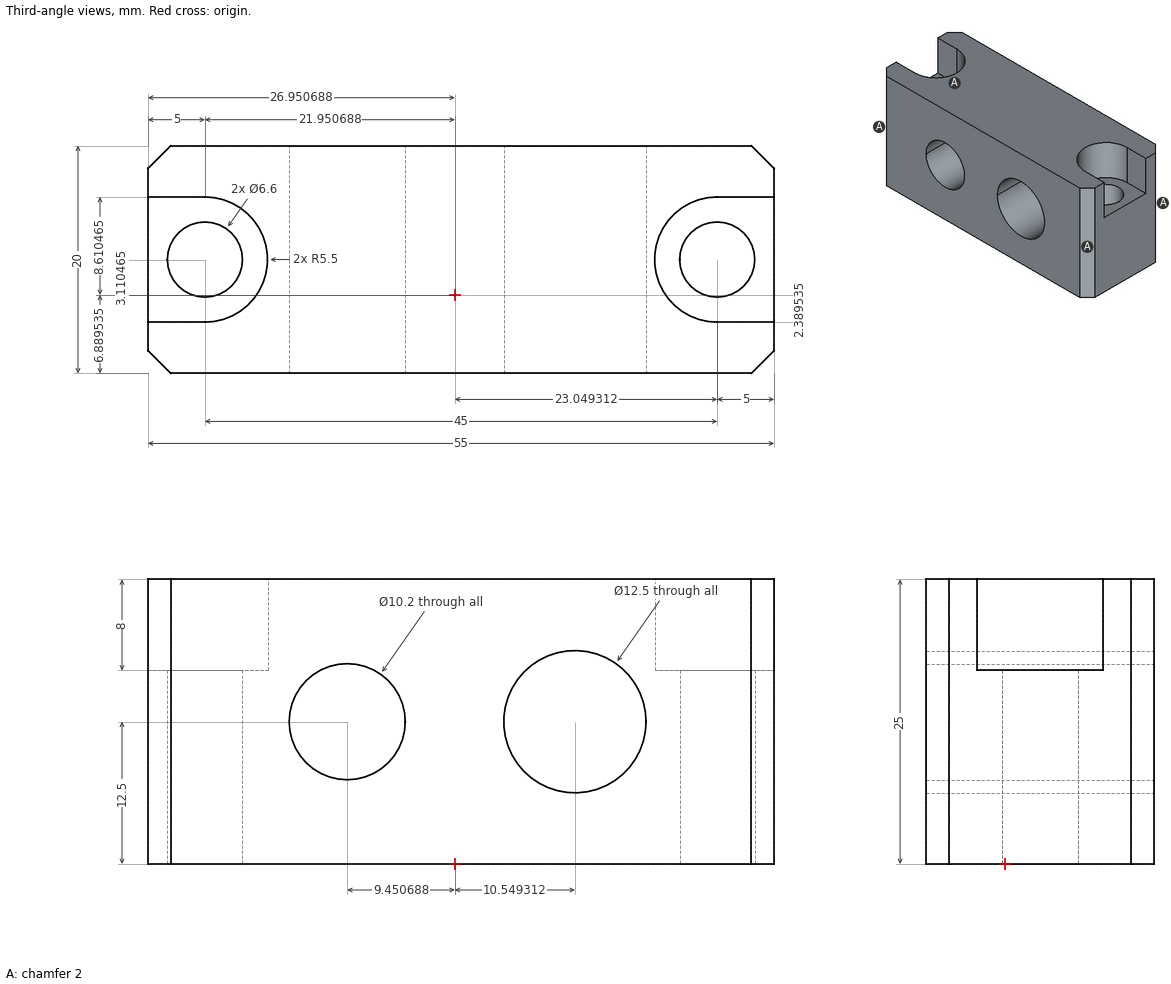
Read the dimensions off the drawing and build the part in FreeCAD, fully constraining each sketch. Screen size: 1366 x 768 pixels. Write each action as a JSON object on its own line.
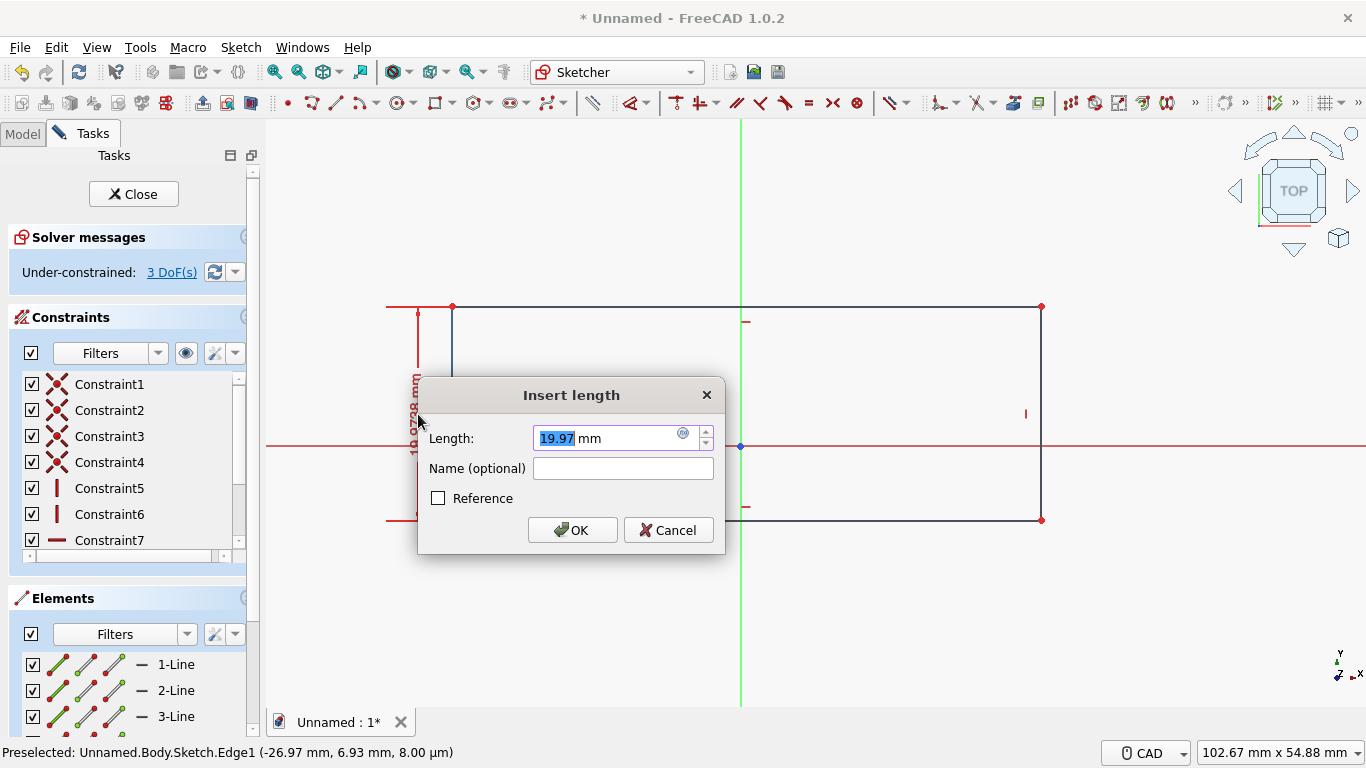
{"action": "type", "text": "20"}
{"action": "key", "text": "Return"}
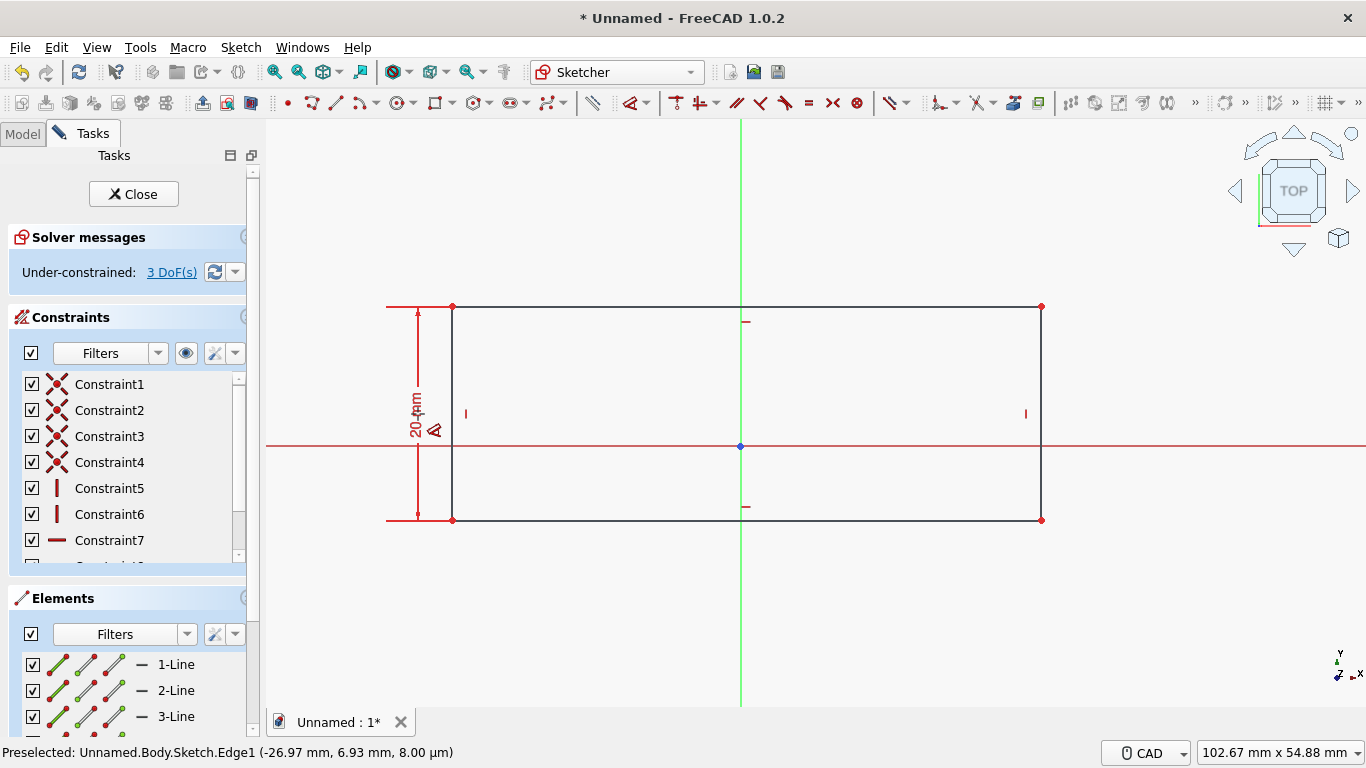
{"action": "left_click", "coordinate": [629, 521]}
{"action": "left_click", "coordinate": [611, 555]}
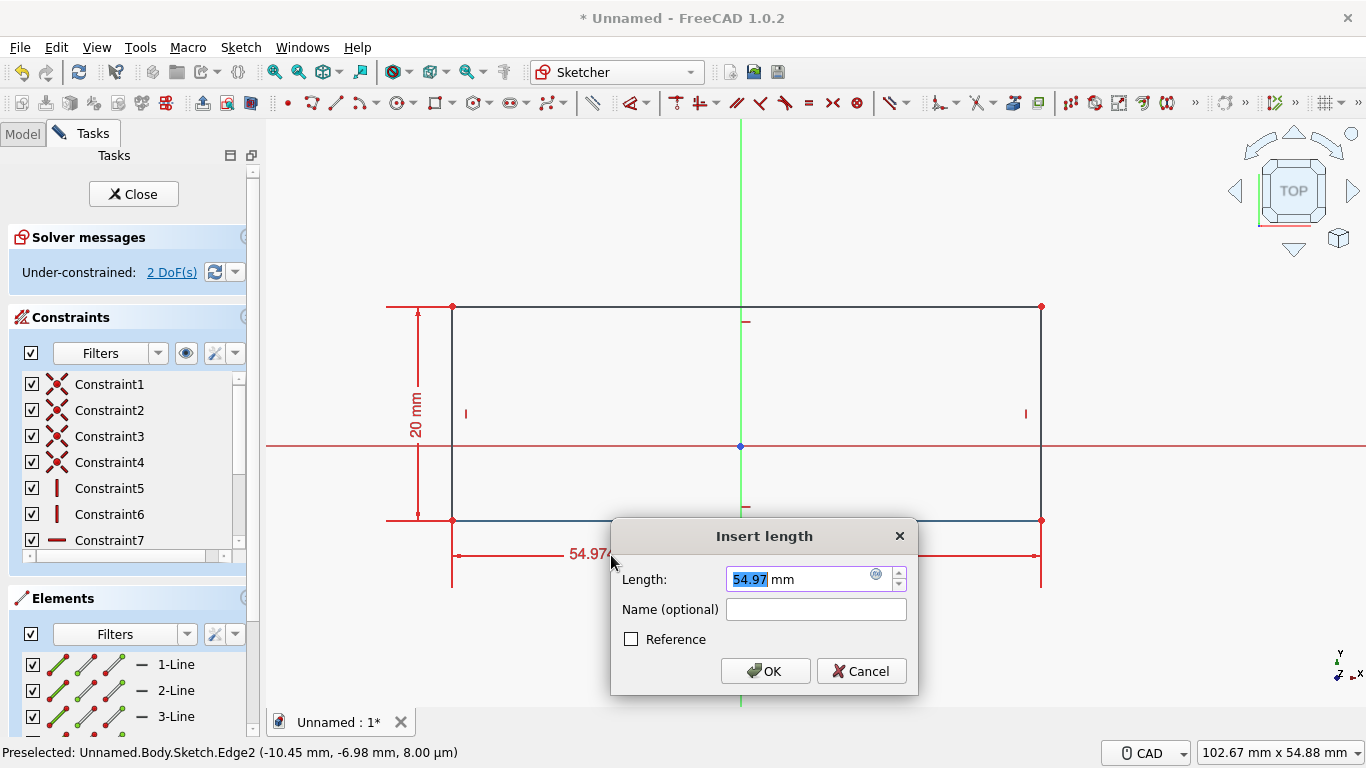
{"action": "type", "text": "55"}
{"action": "key", "text": "Return"}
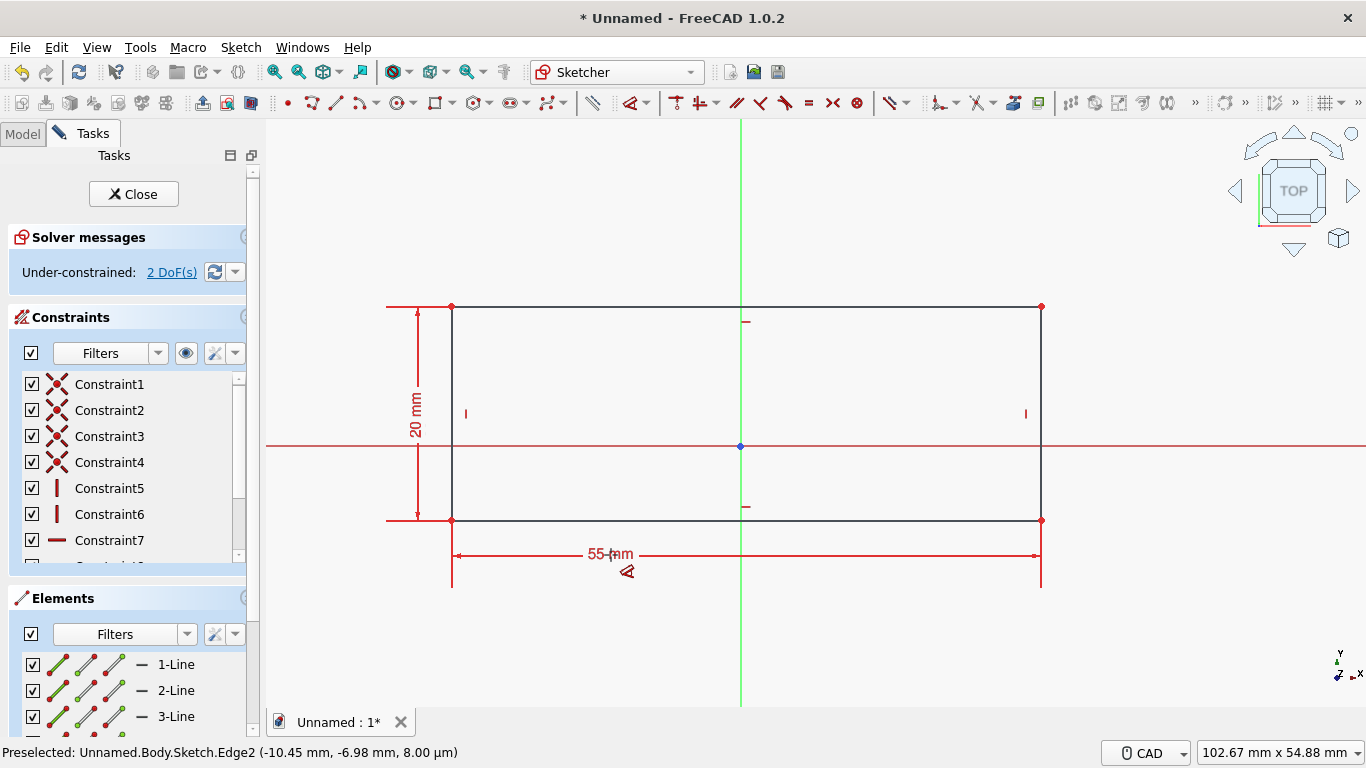
{"action": "left_click", "coordinate": [452, 521]}
{"action": "left_click", "coordinate": [418, 484]}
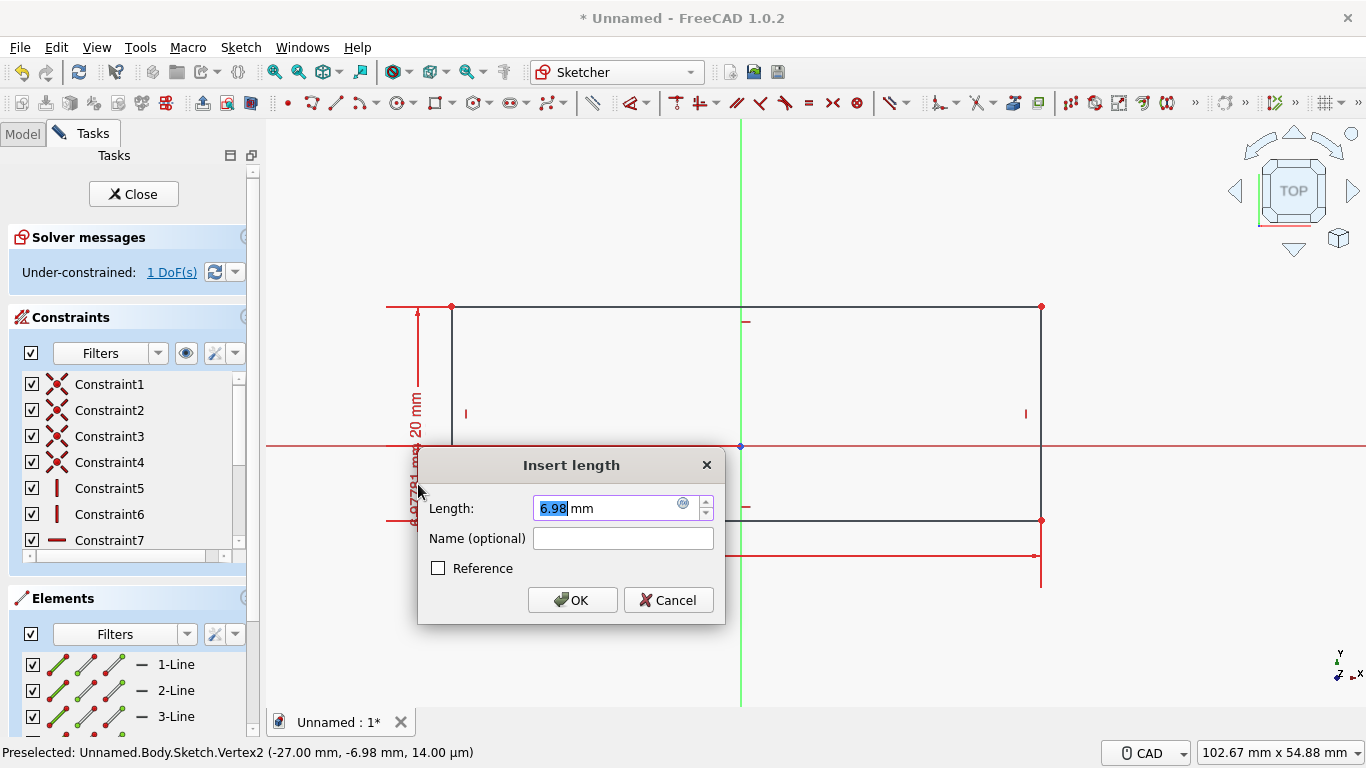
{"action": "type", "text": "6.889535"}
{"action": "key", "text": "Return"}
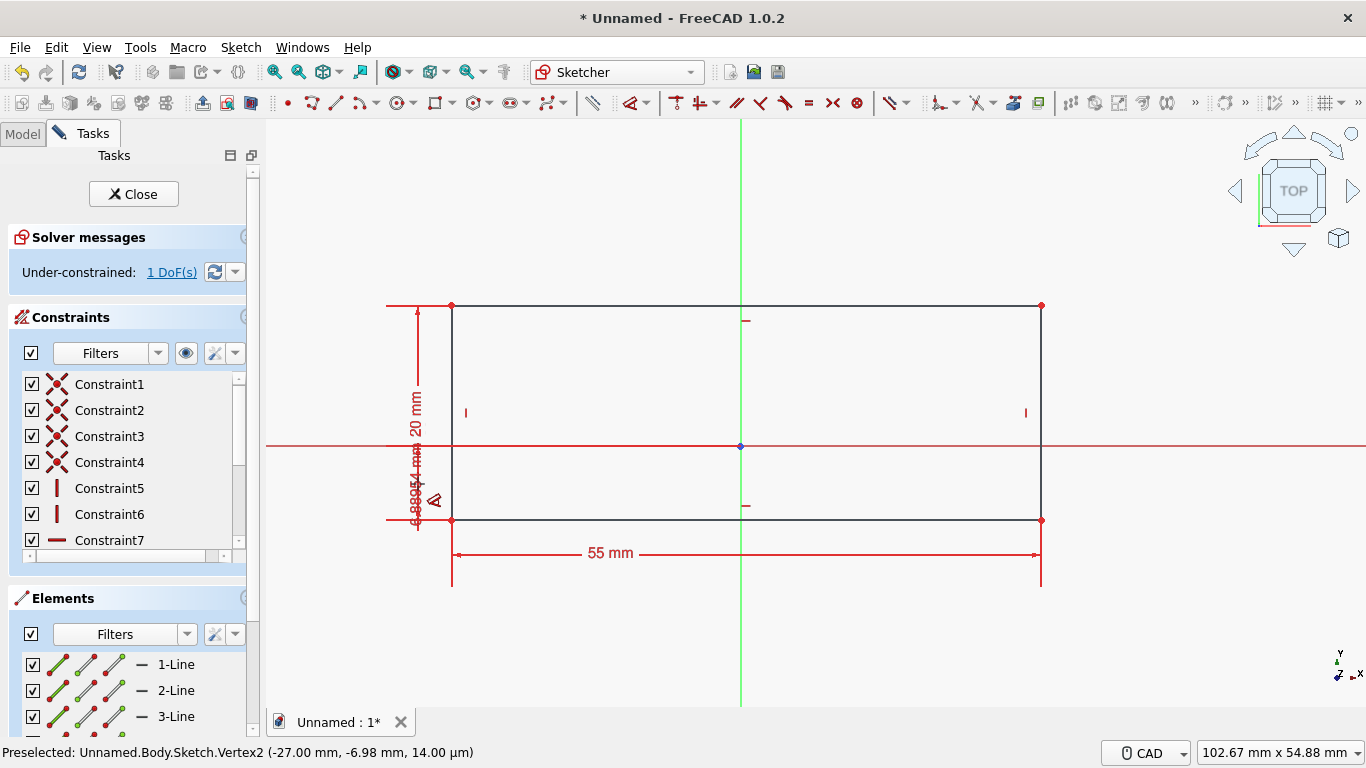
{"action": "left_click", "coordinate": [452, 306]}
{"action": "left_click", "coordinate": [596, 272]}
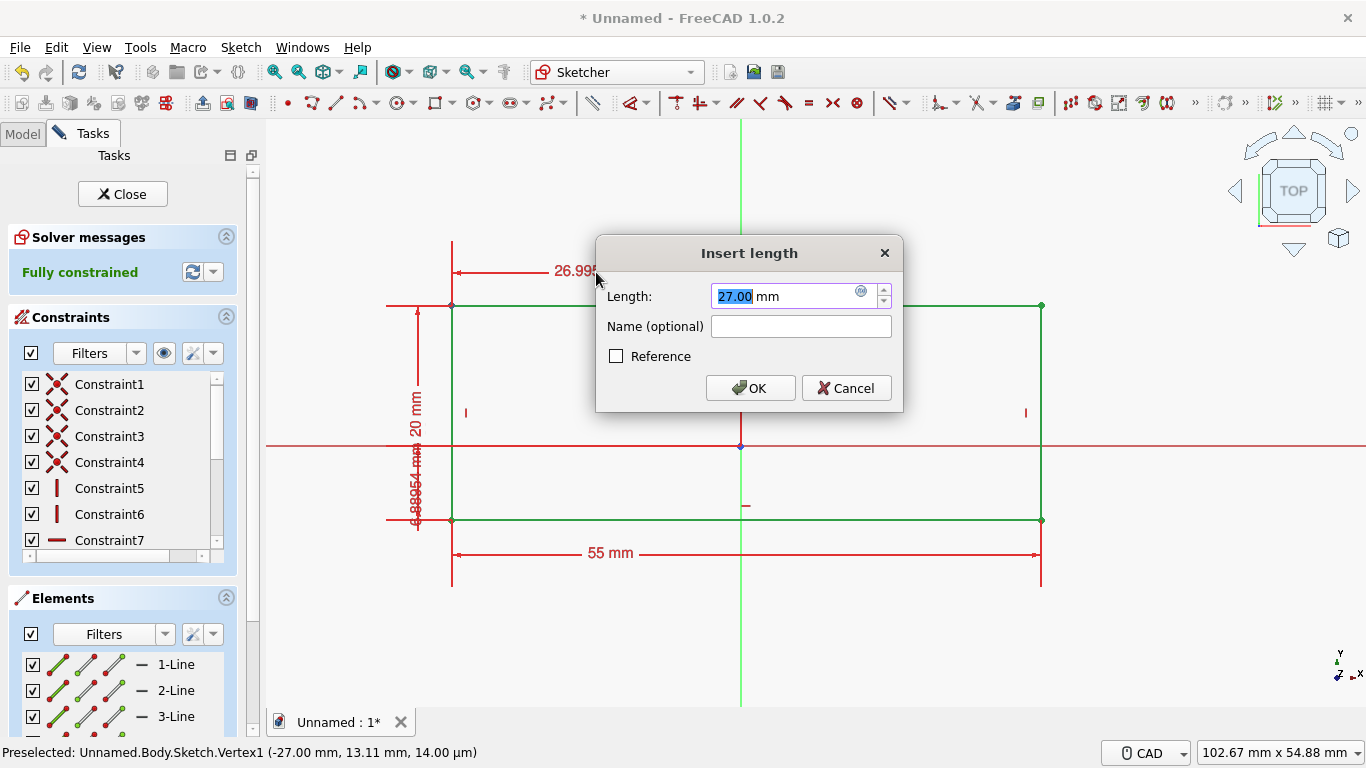
{"action": "type", "text": "26.950688"}
{"action": "key", "text": "Return"}
{"action": "key", "text": "Escape"}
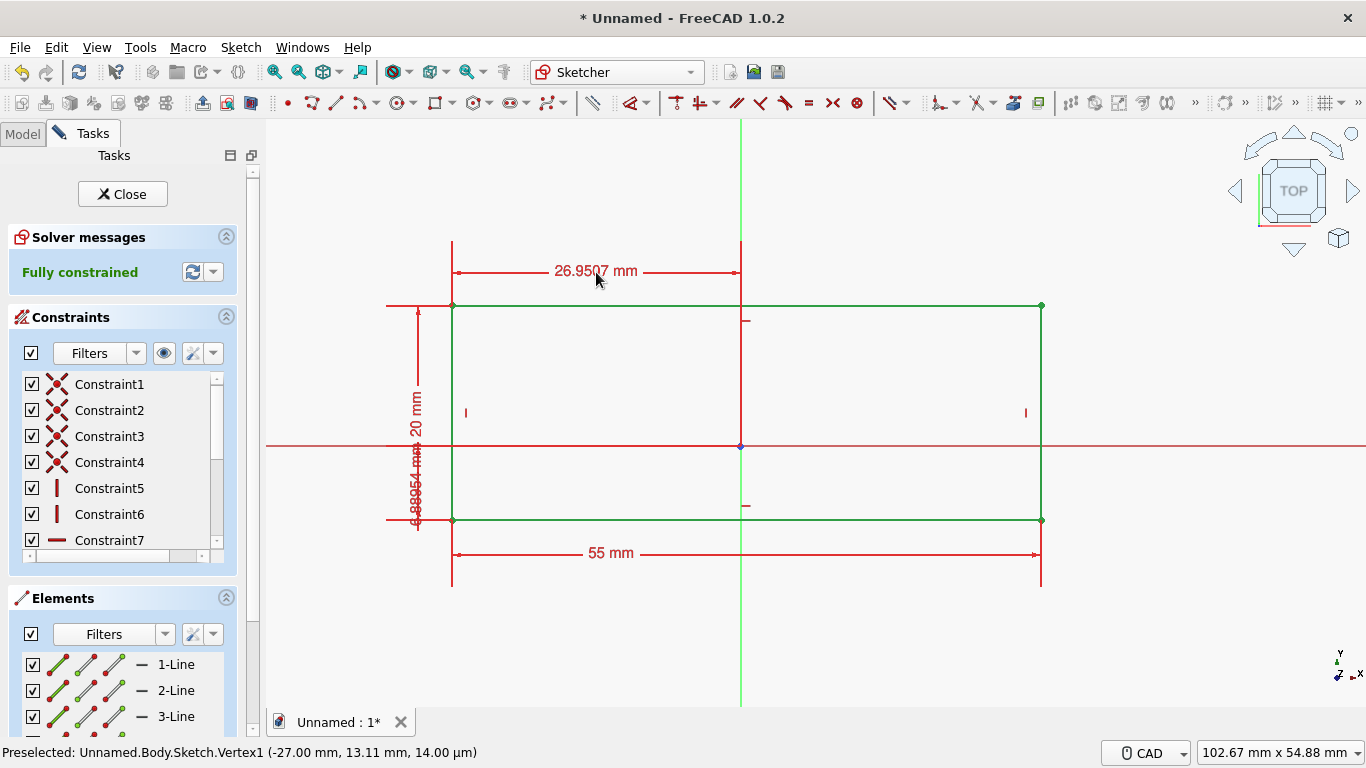
{"action": "left_click", "coordinate": [123, 194]}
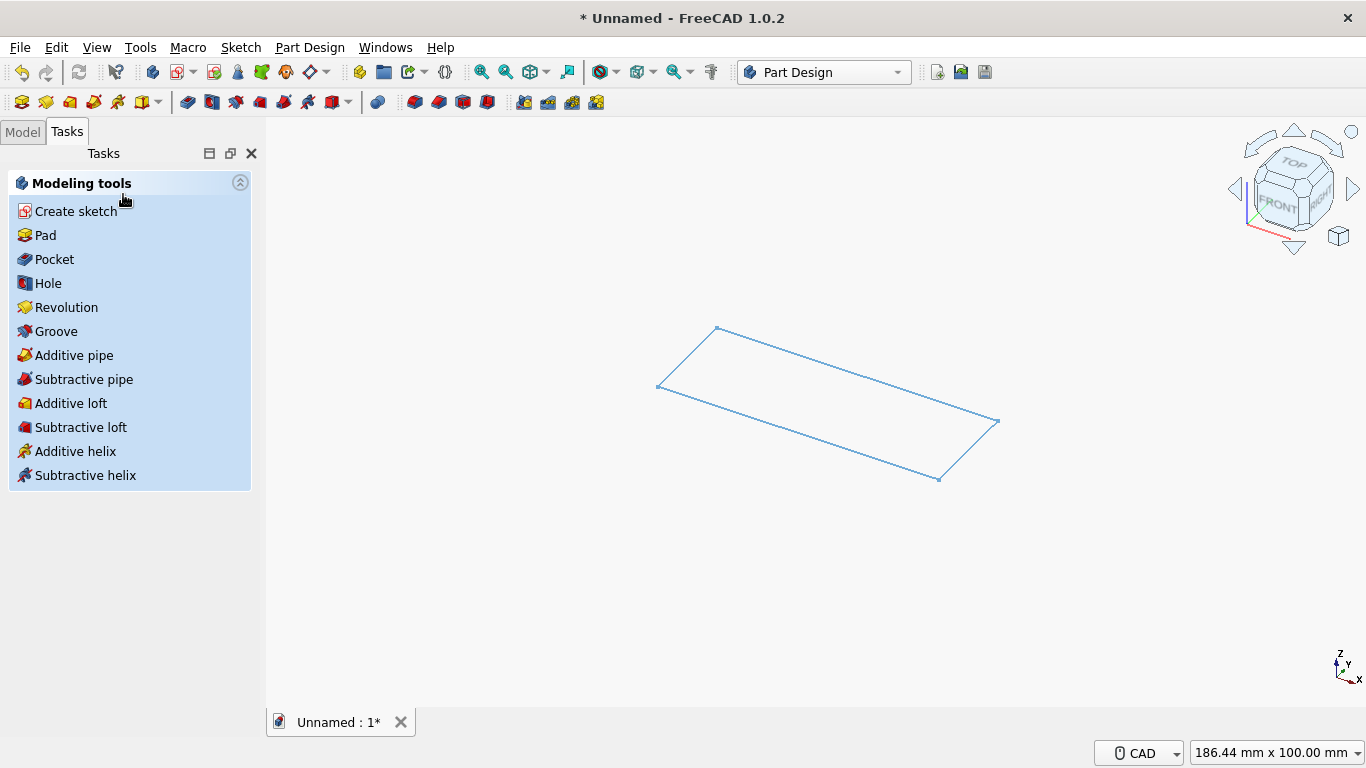
{"action": "left_click", "coordinate": [22, 102]}